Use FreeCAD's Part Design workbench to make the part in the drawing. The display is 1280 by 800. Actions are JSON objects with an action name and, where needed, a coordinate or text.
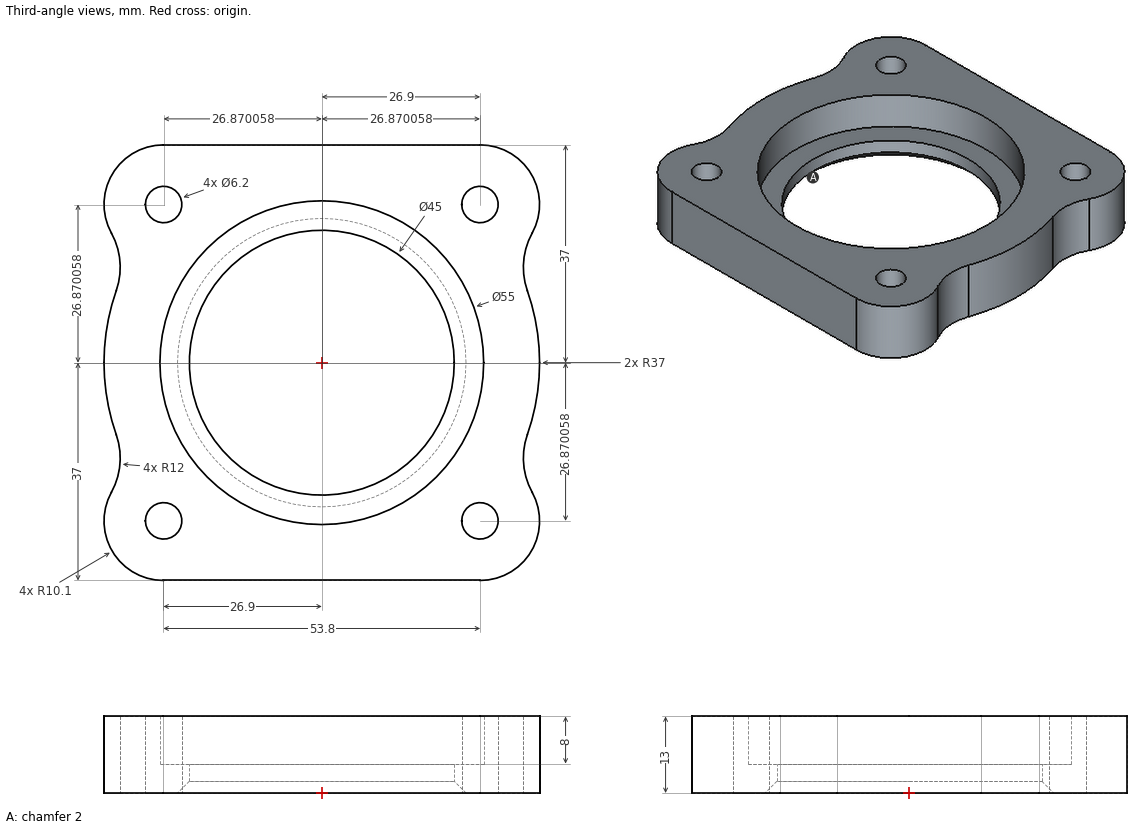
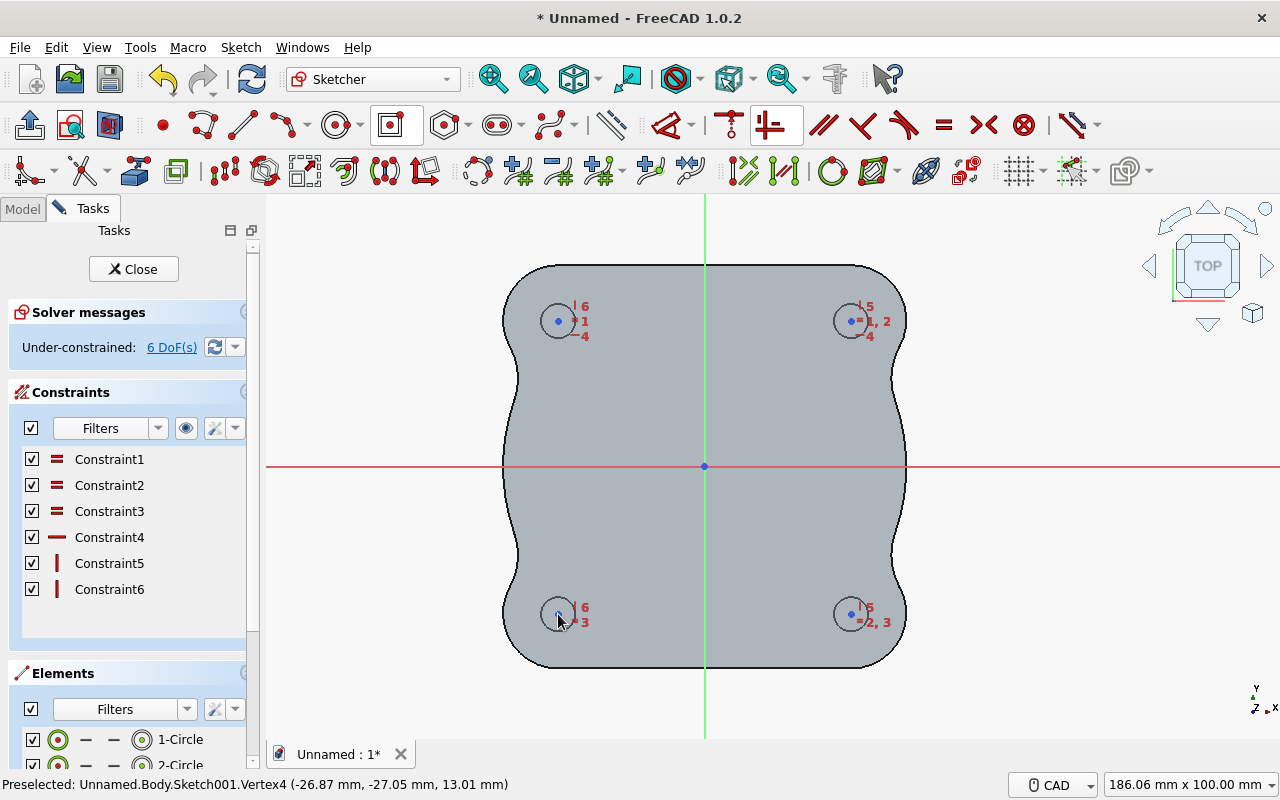
{"action": "left_click", "coordinate": [851, 614]}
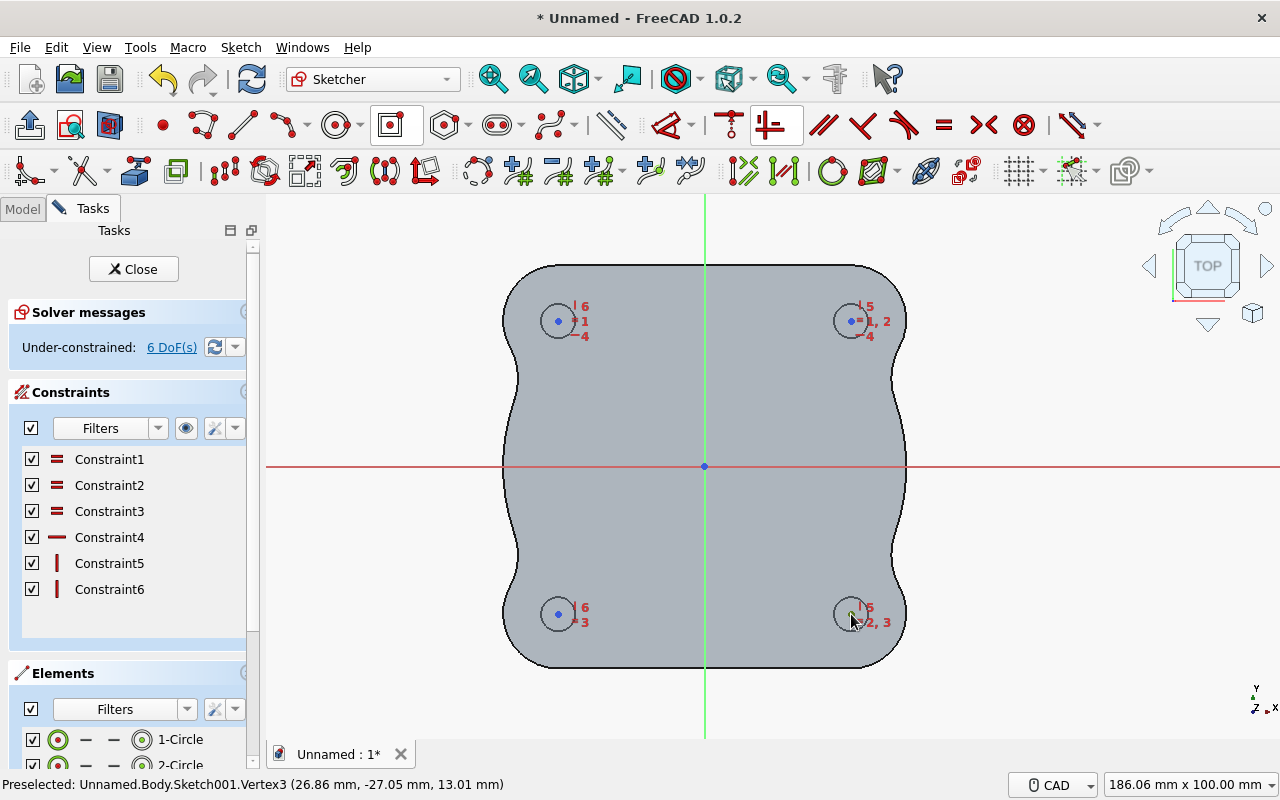
{"action": "left_click", "coordinate": [558, 614]}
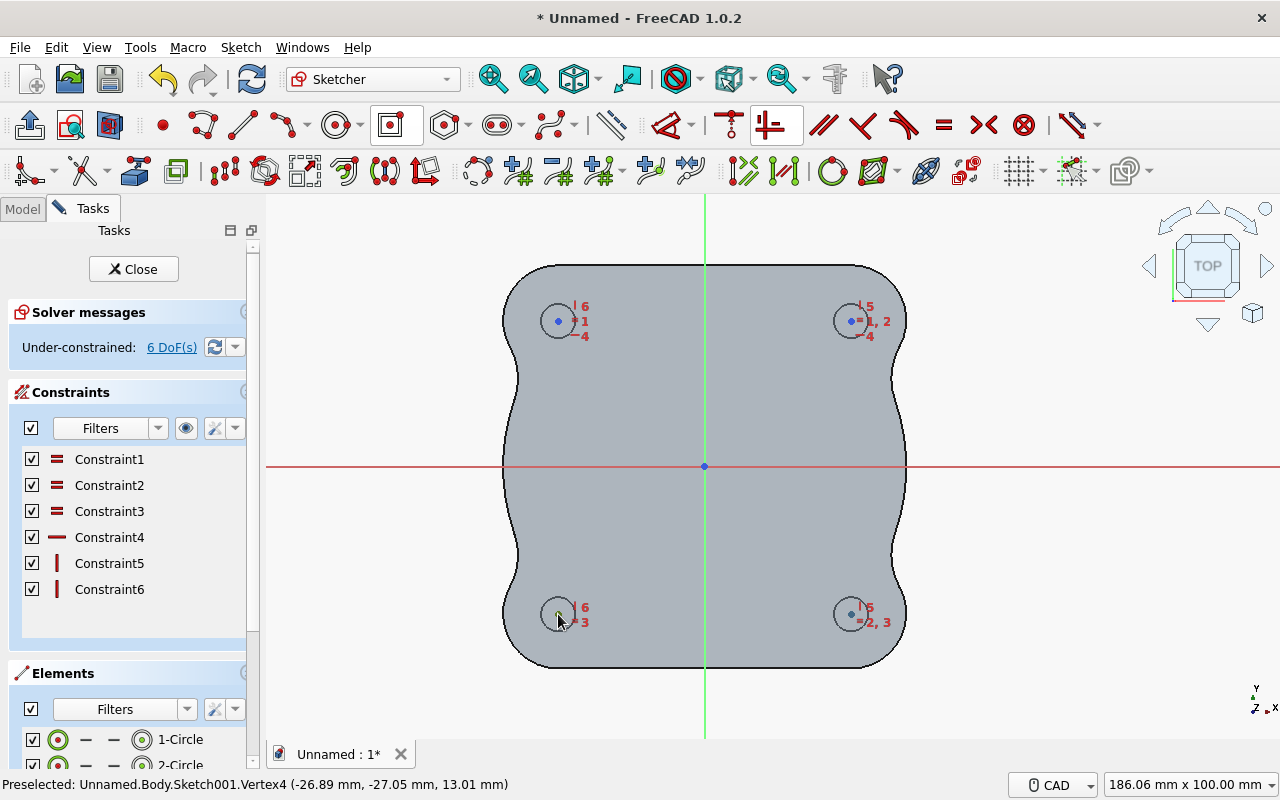
{"action": "key", "text": "h"}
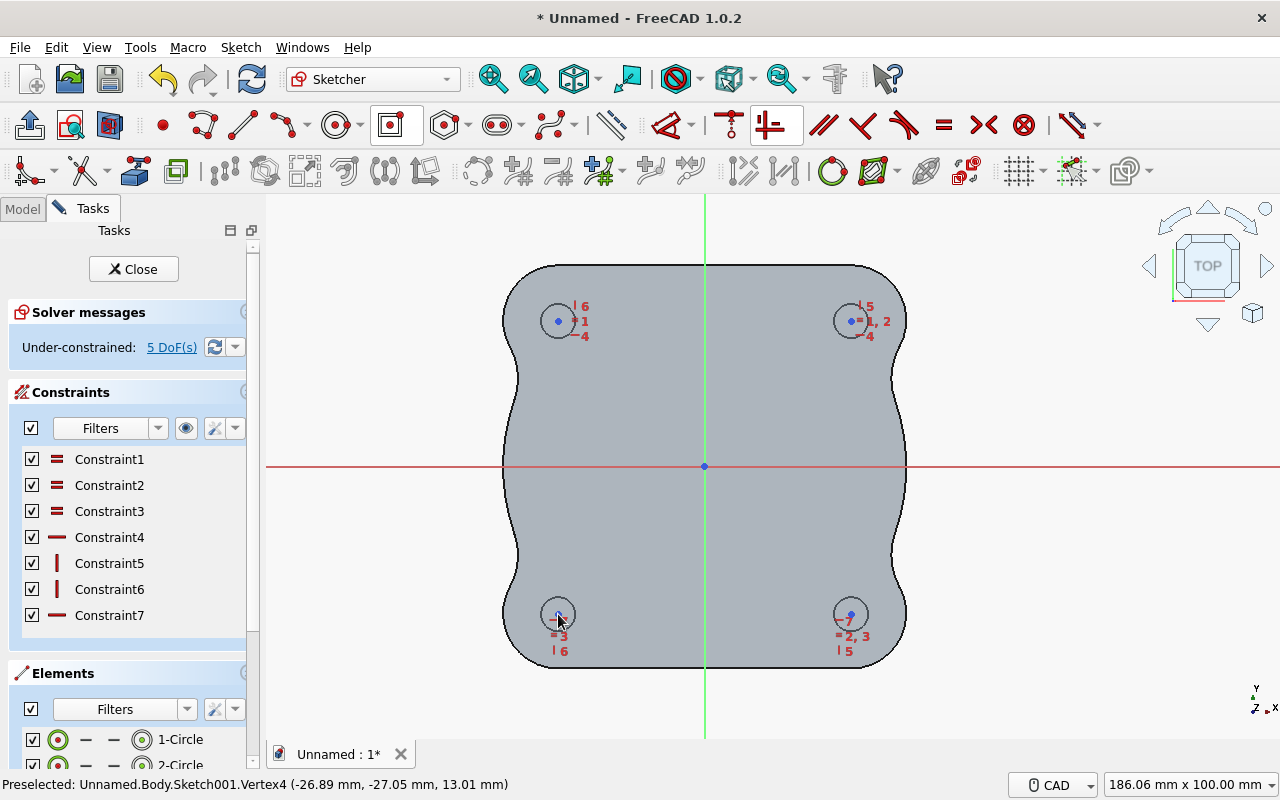
{"action": "key", "text": "d"}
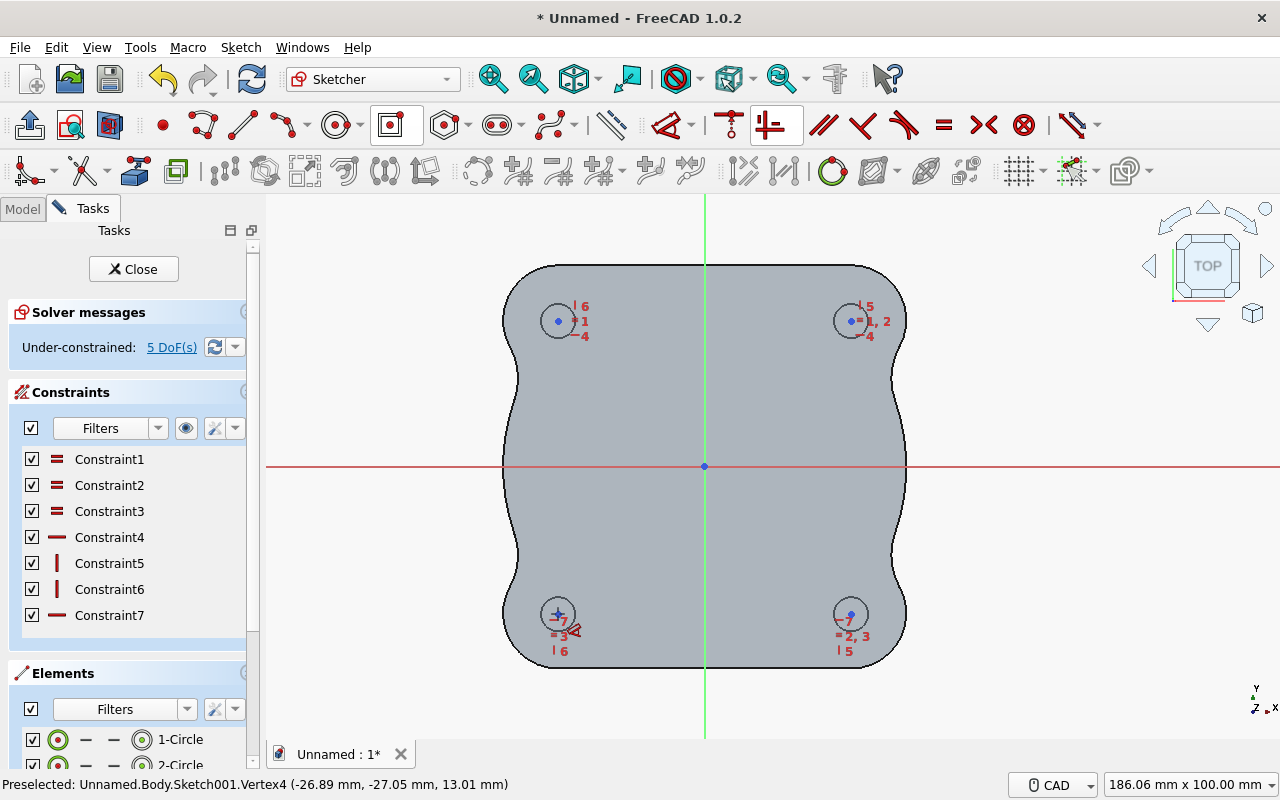
{"action": "left_click", "coordinate": [570, 309]}
{"action": "left_click", "coordinate": [592, 286]}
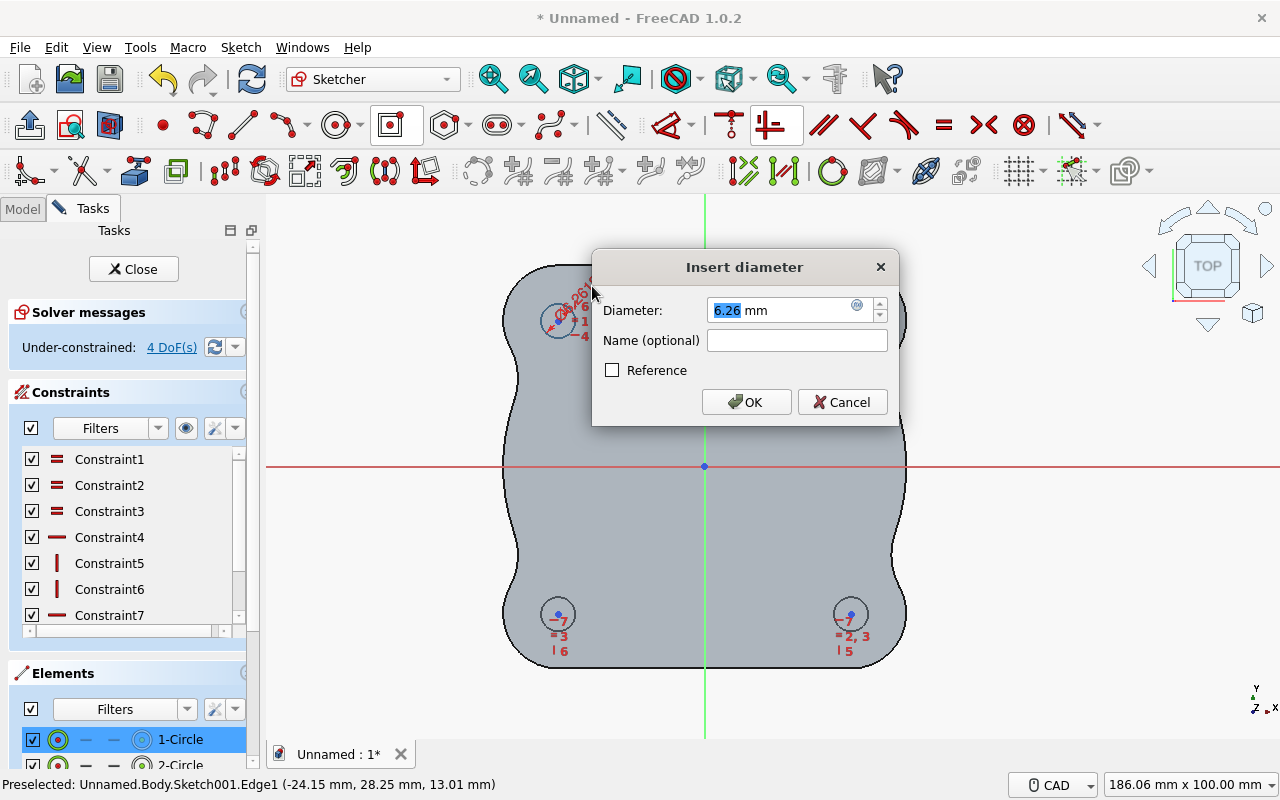
{"action": "type", "text": "6.2"}
{"action": "key", "text": "Return"}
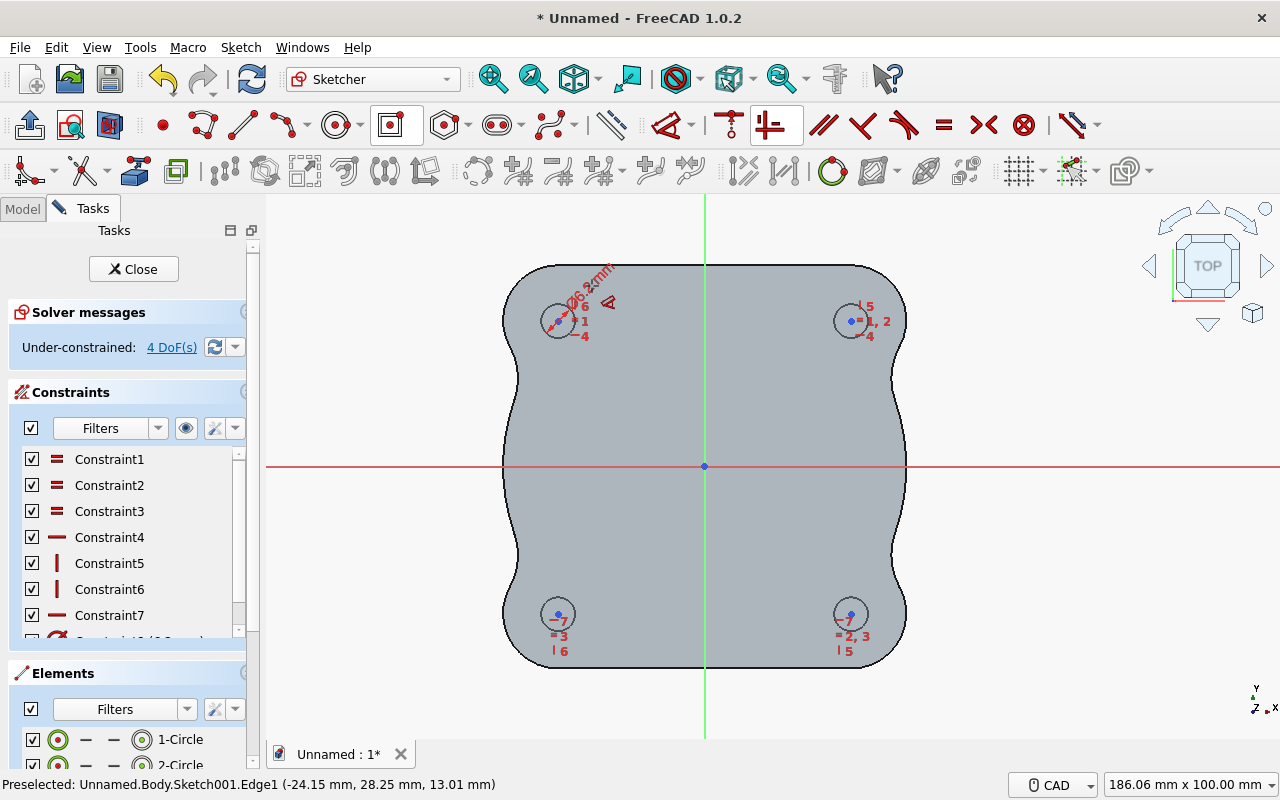
{"action": "left_click", "coordinate": [558, 321]}
{"action": "left_click", "coordinate": [665, 287]}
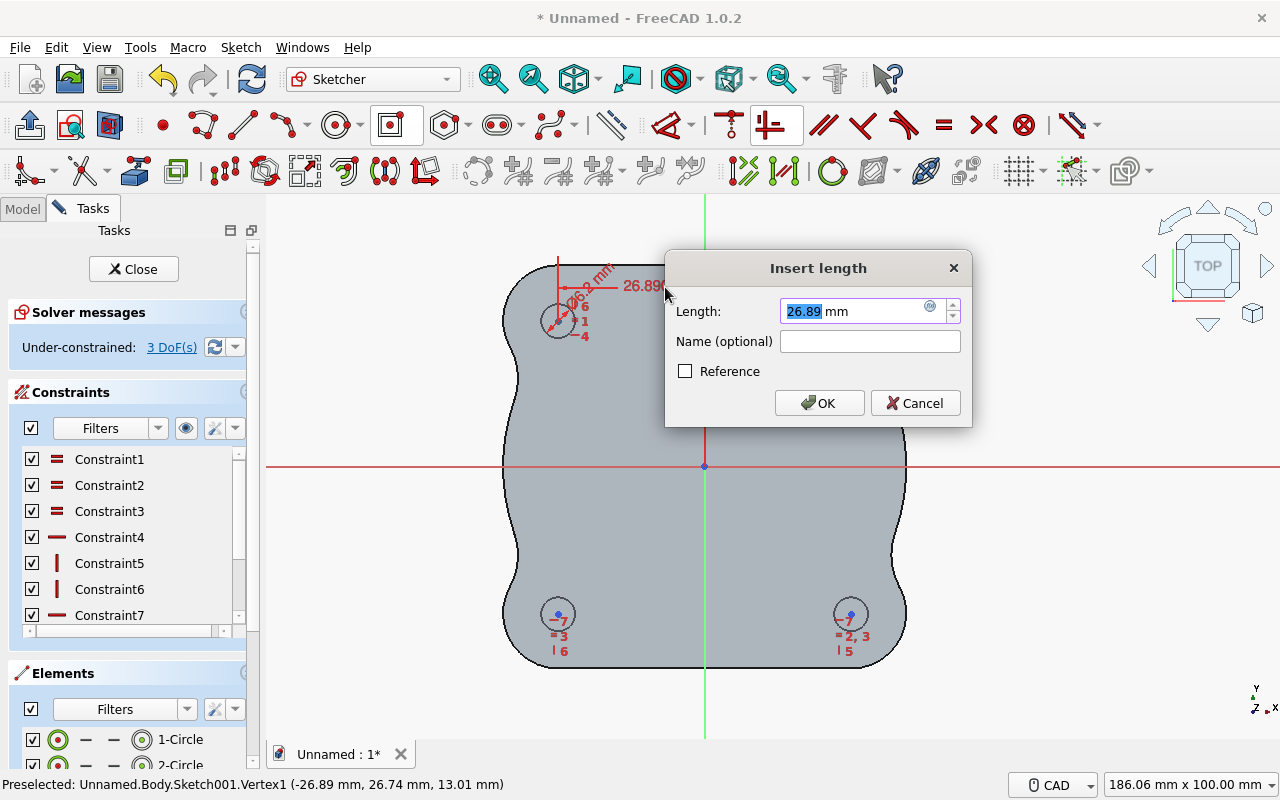
{"action": "type", "text": "26.870058"}
{"action": "key", "text": "Return"}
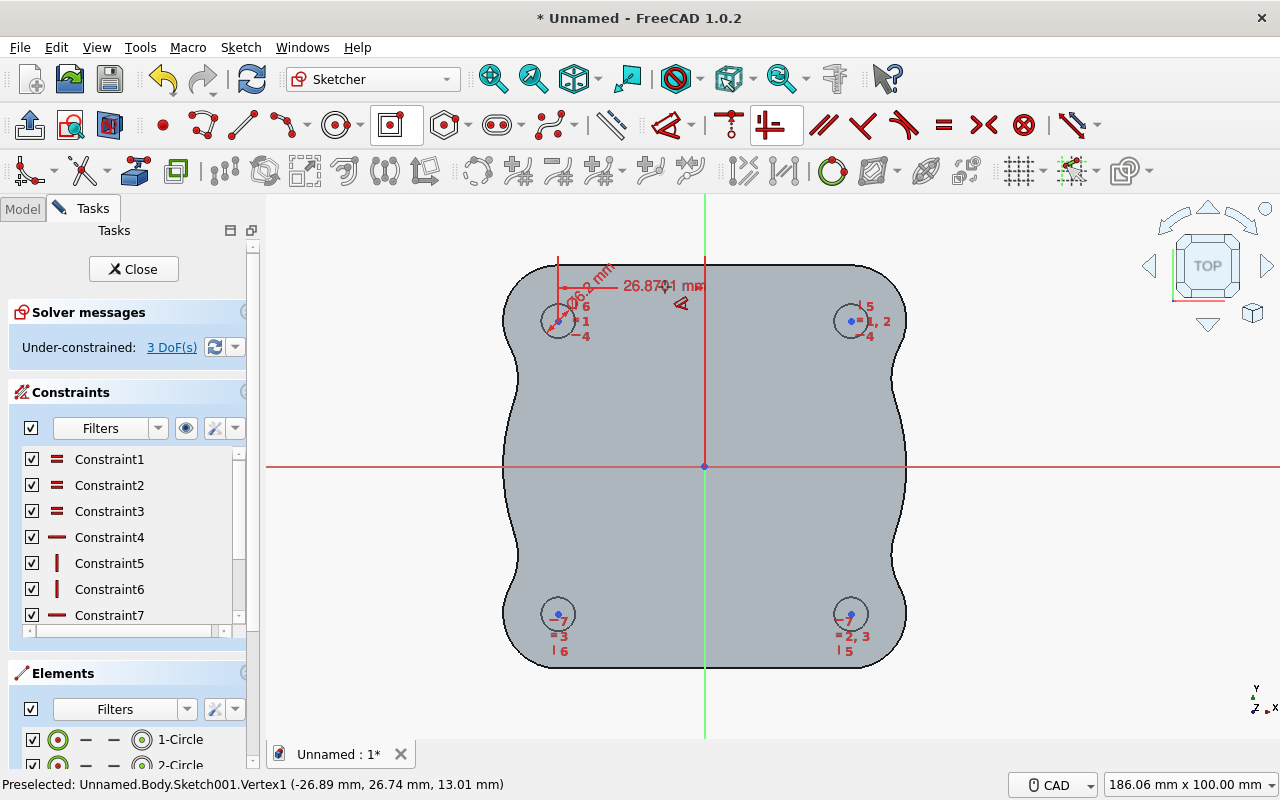
{"action": "left_click", "coordinate": [558, 321]}
{"action": "left_click", "coordinate": [524, 394]}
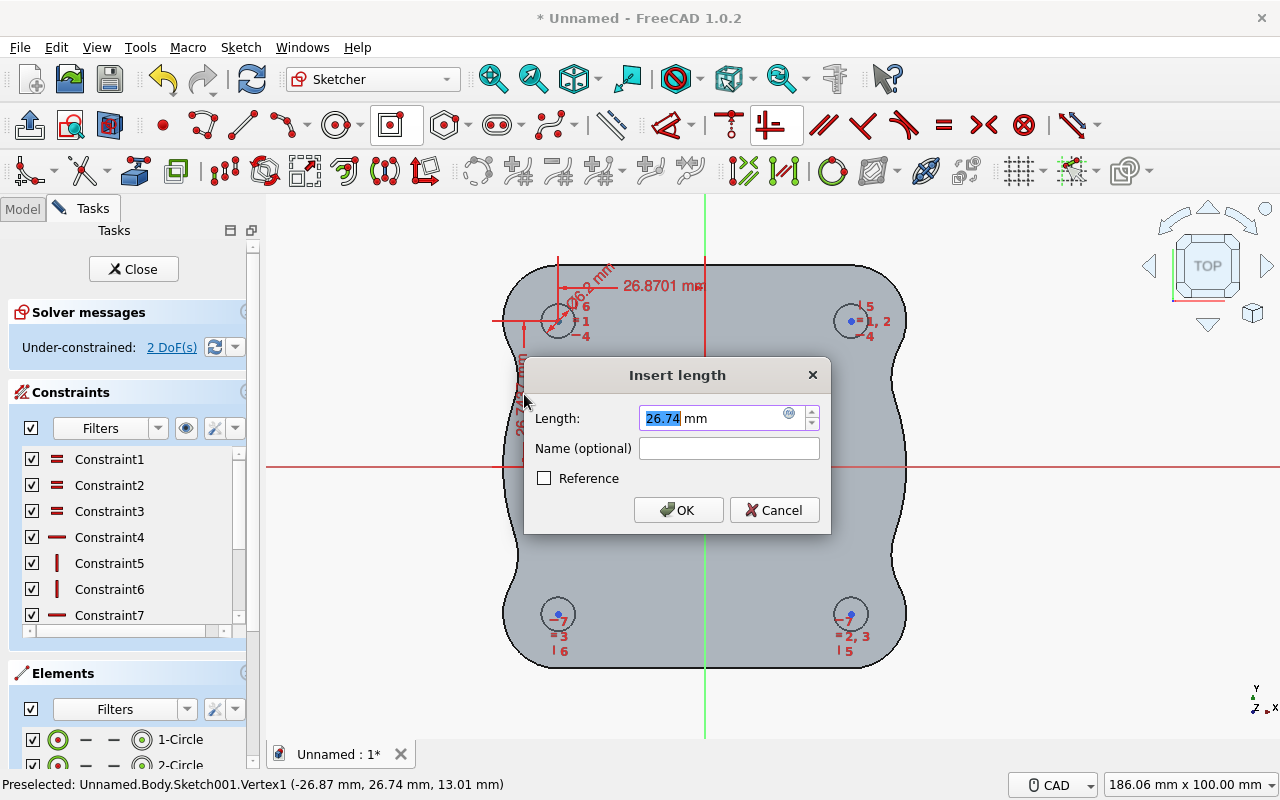
{"action": "type", "text": "26.870058"}
{"action": "key", "text": "Return"}